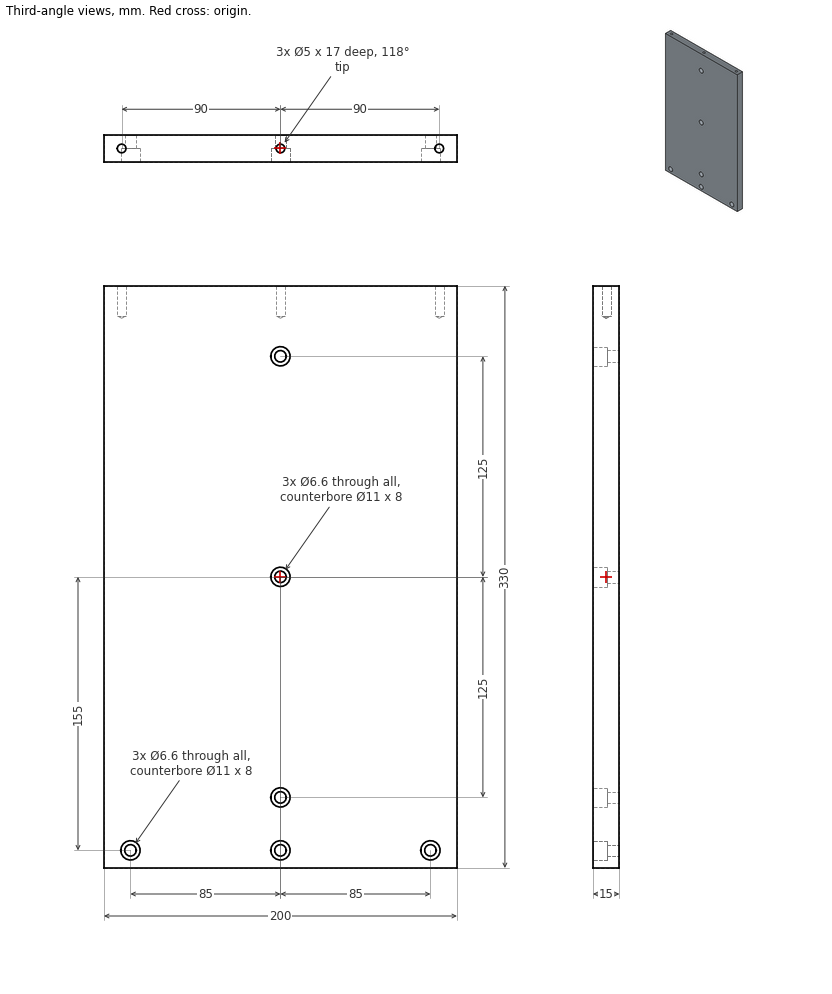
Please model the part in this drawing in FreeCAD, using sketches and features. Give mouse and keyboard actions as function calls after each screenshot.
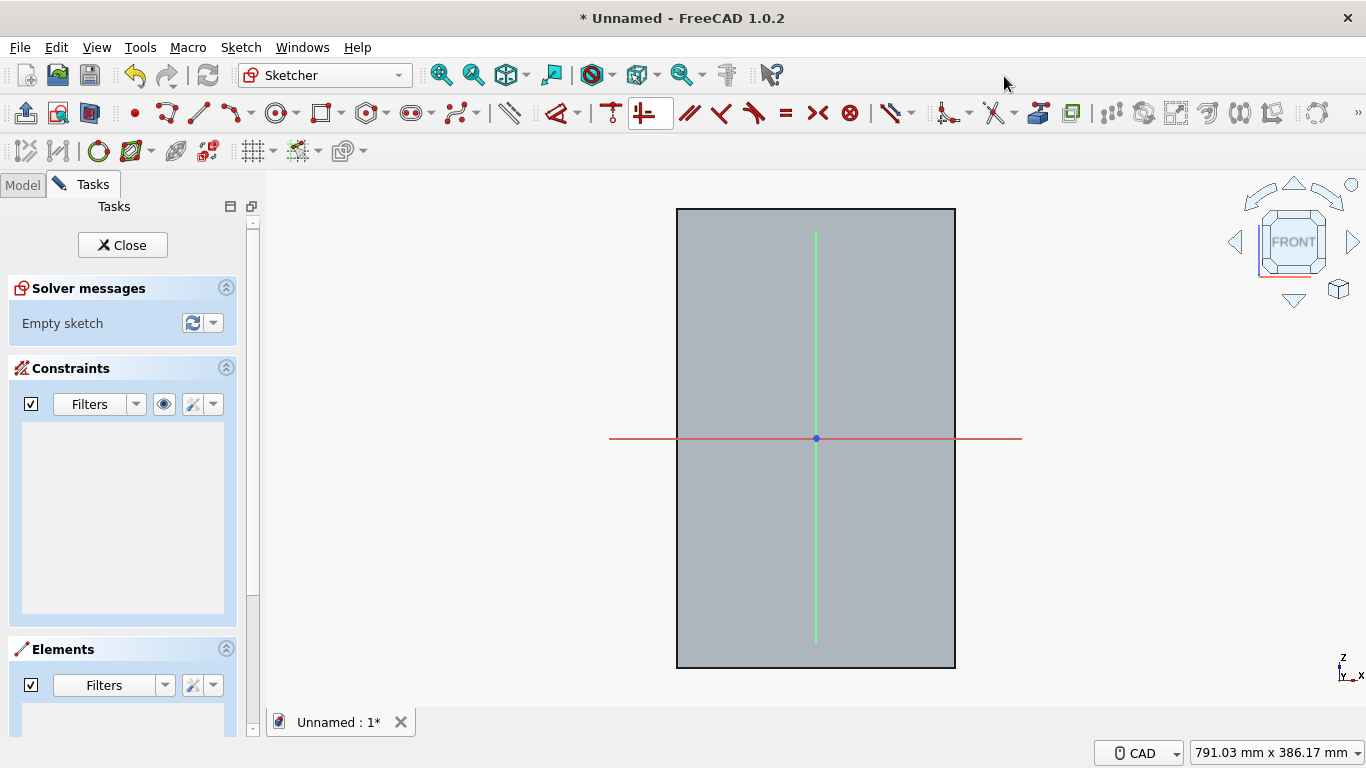
key(g)
key(c)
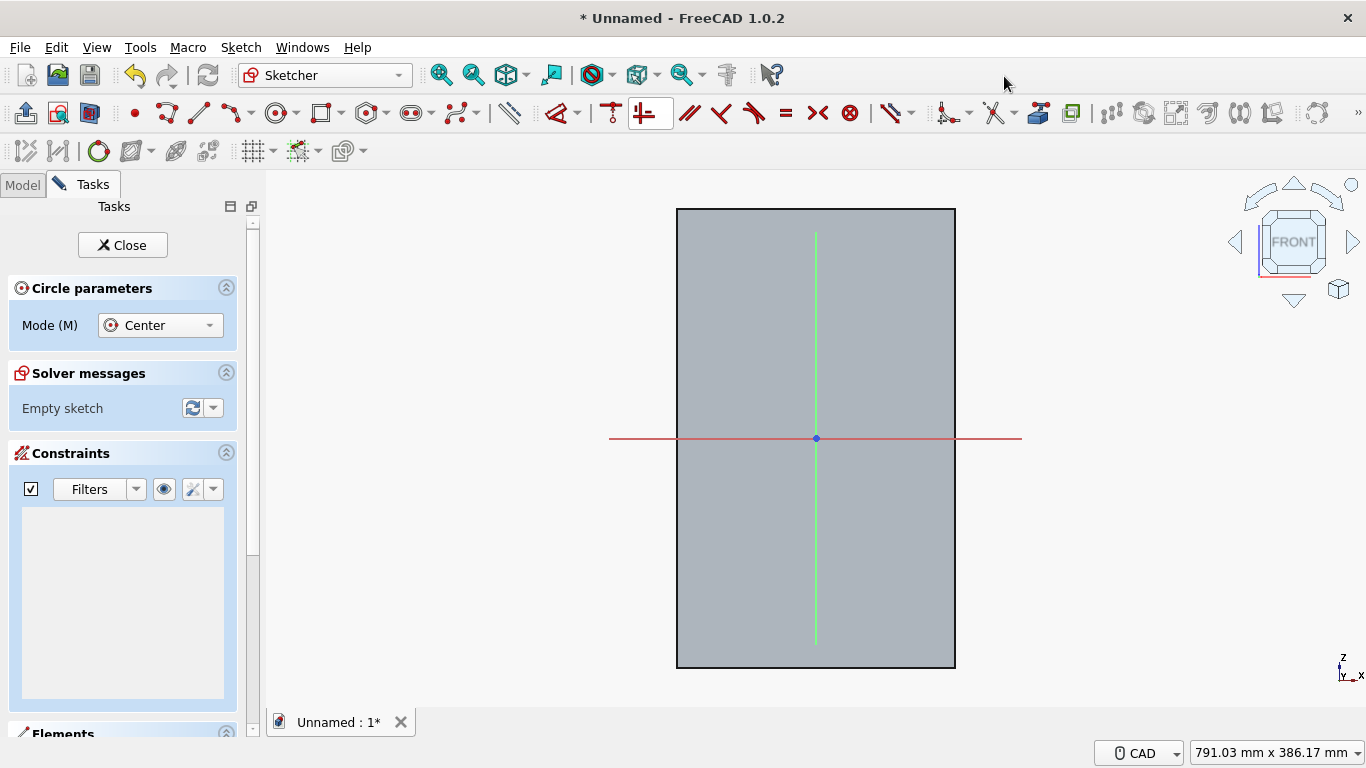
scroll(816, 439, up, 8)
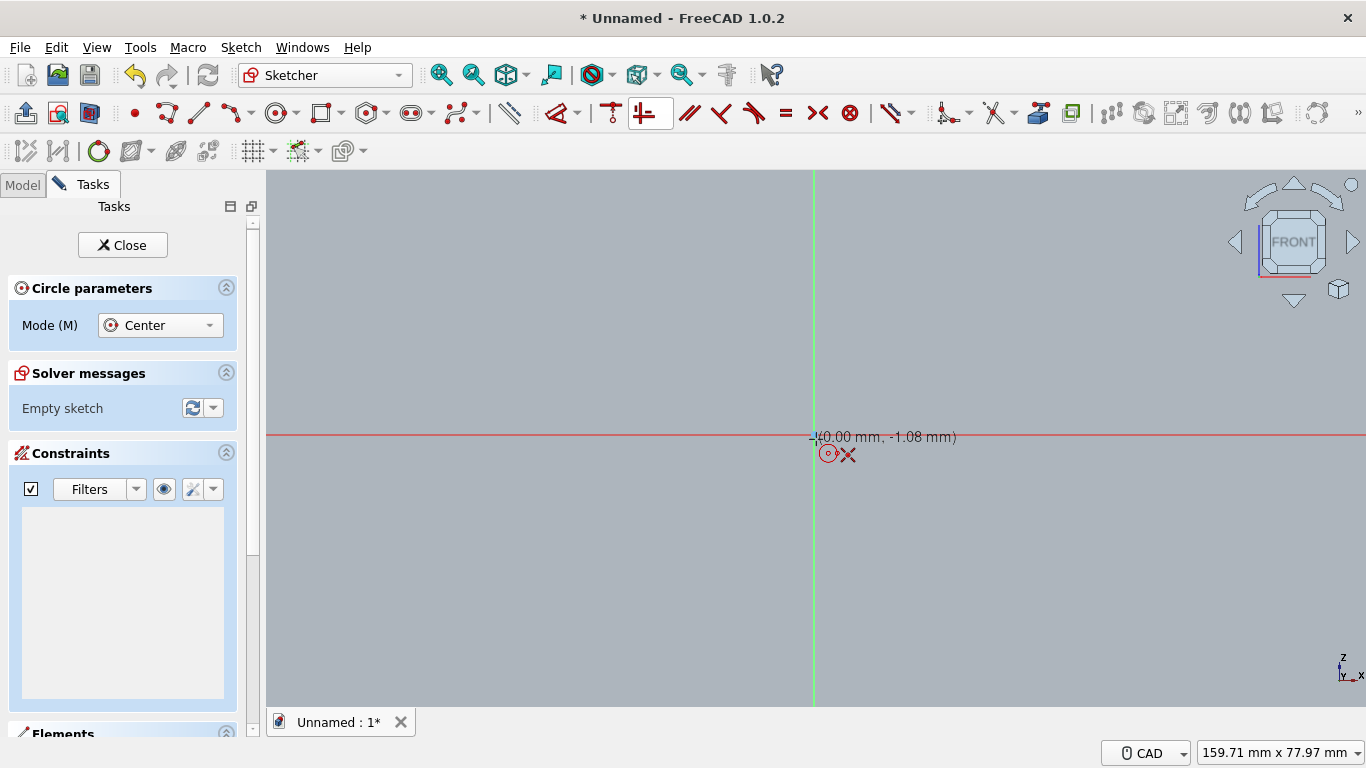
scroll(731, 440, down, 8)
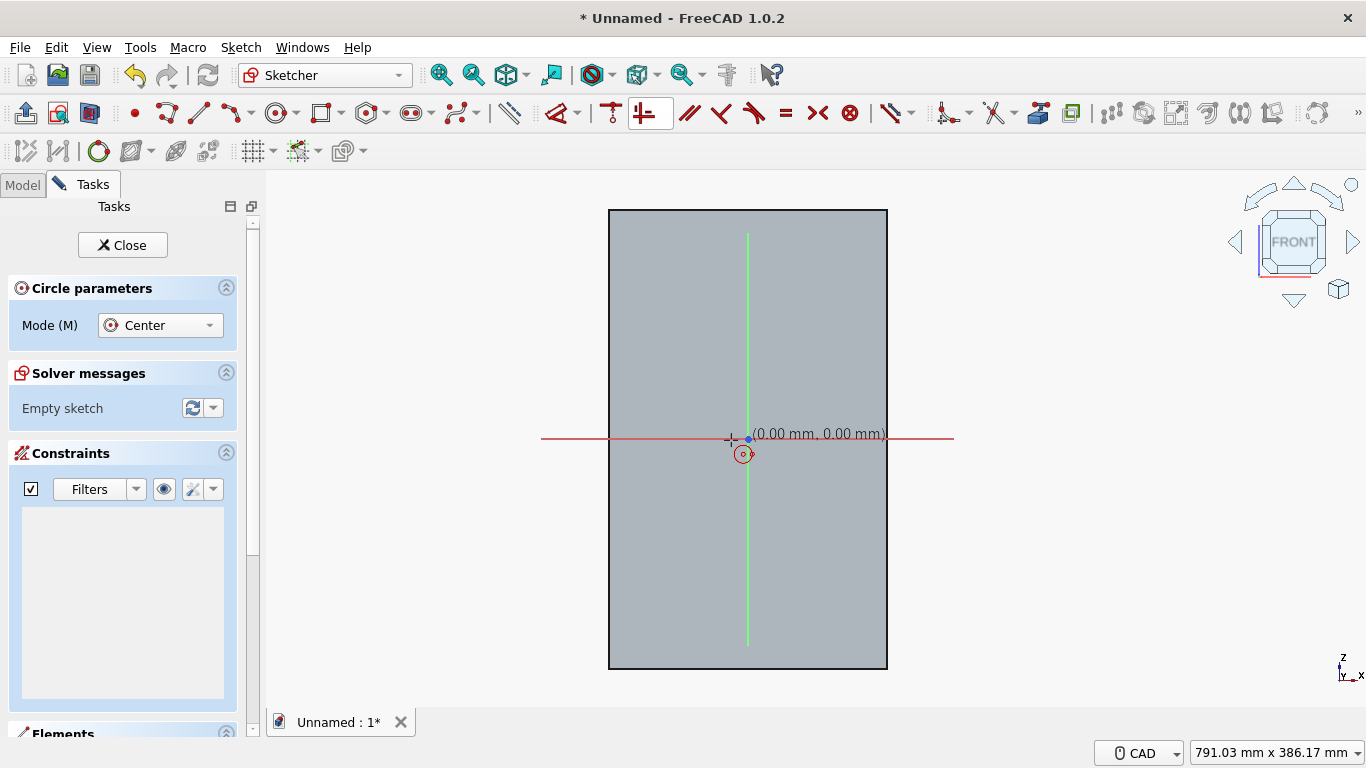
click(748, 439)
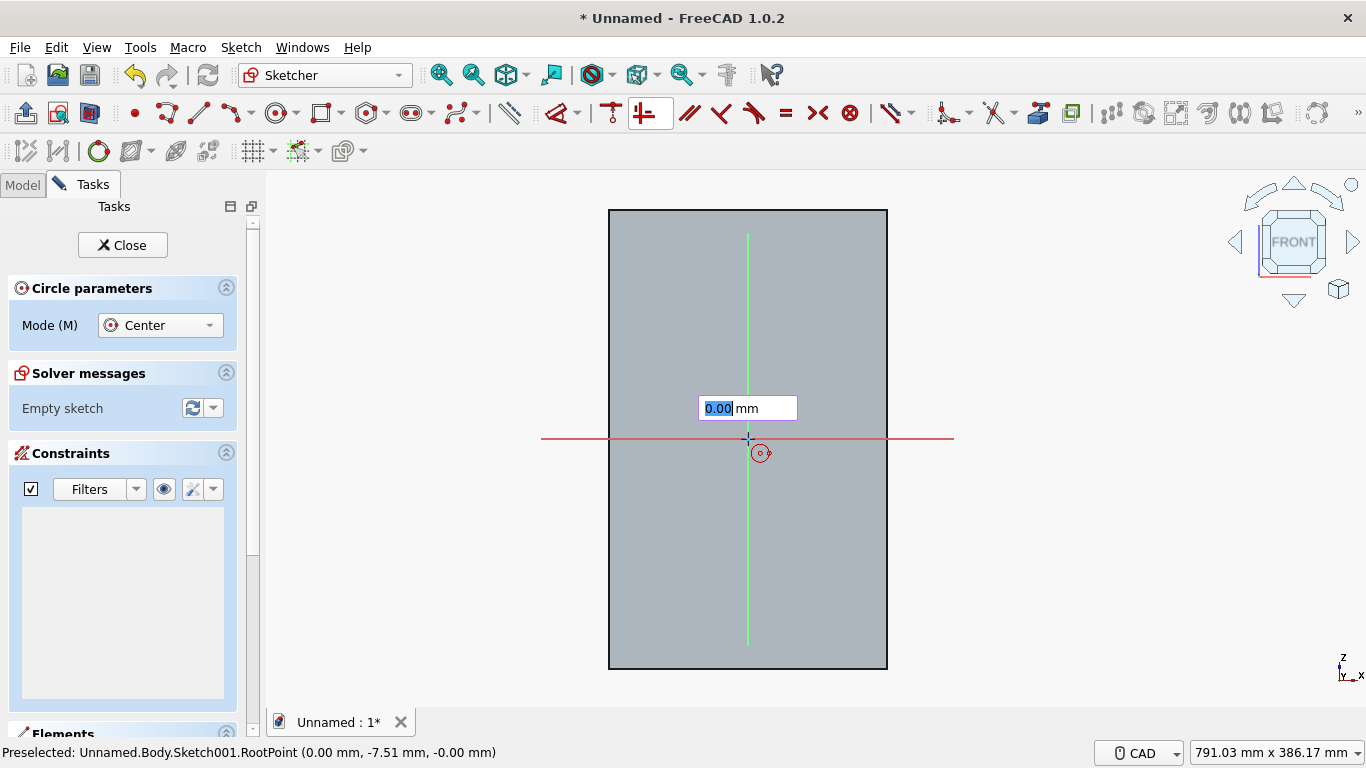
scroll(751, 436, up, 8)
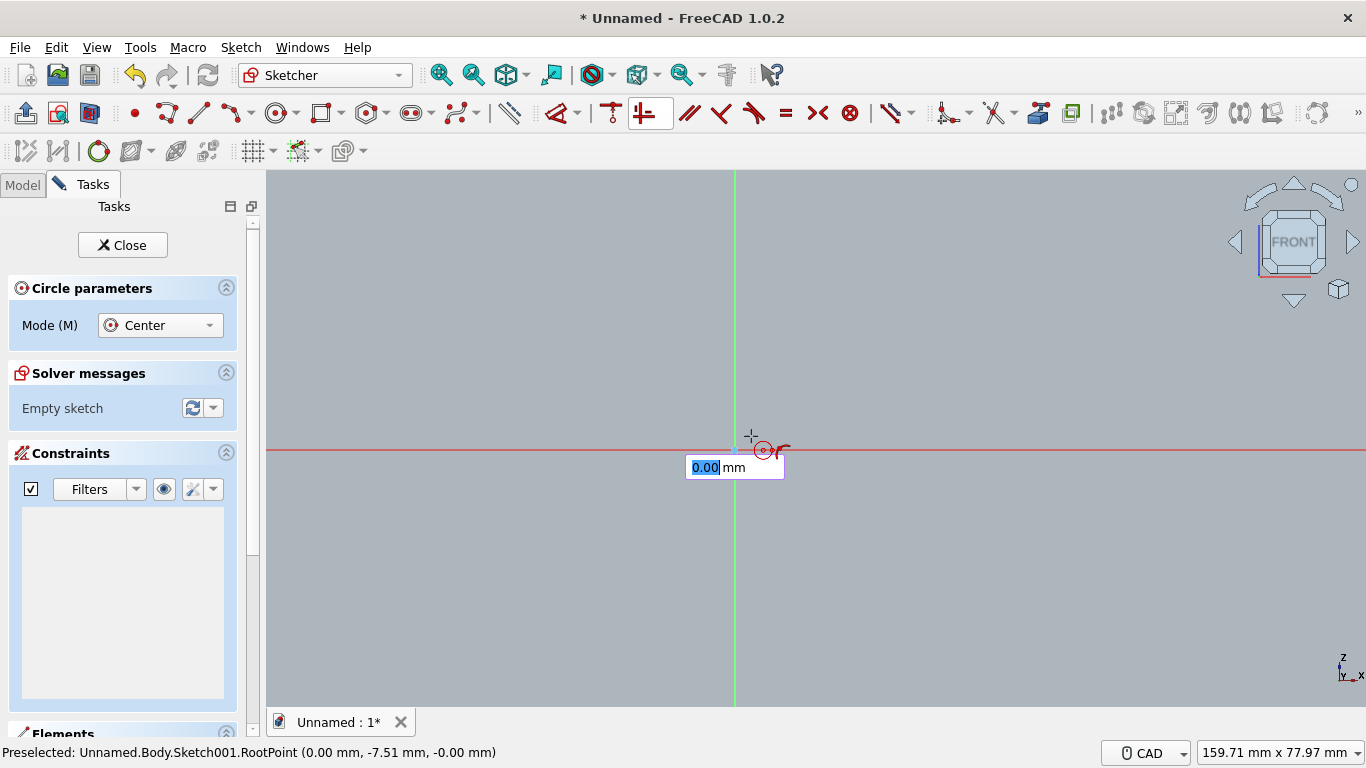
click(751, 434)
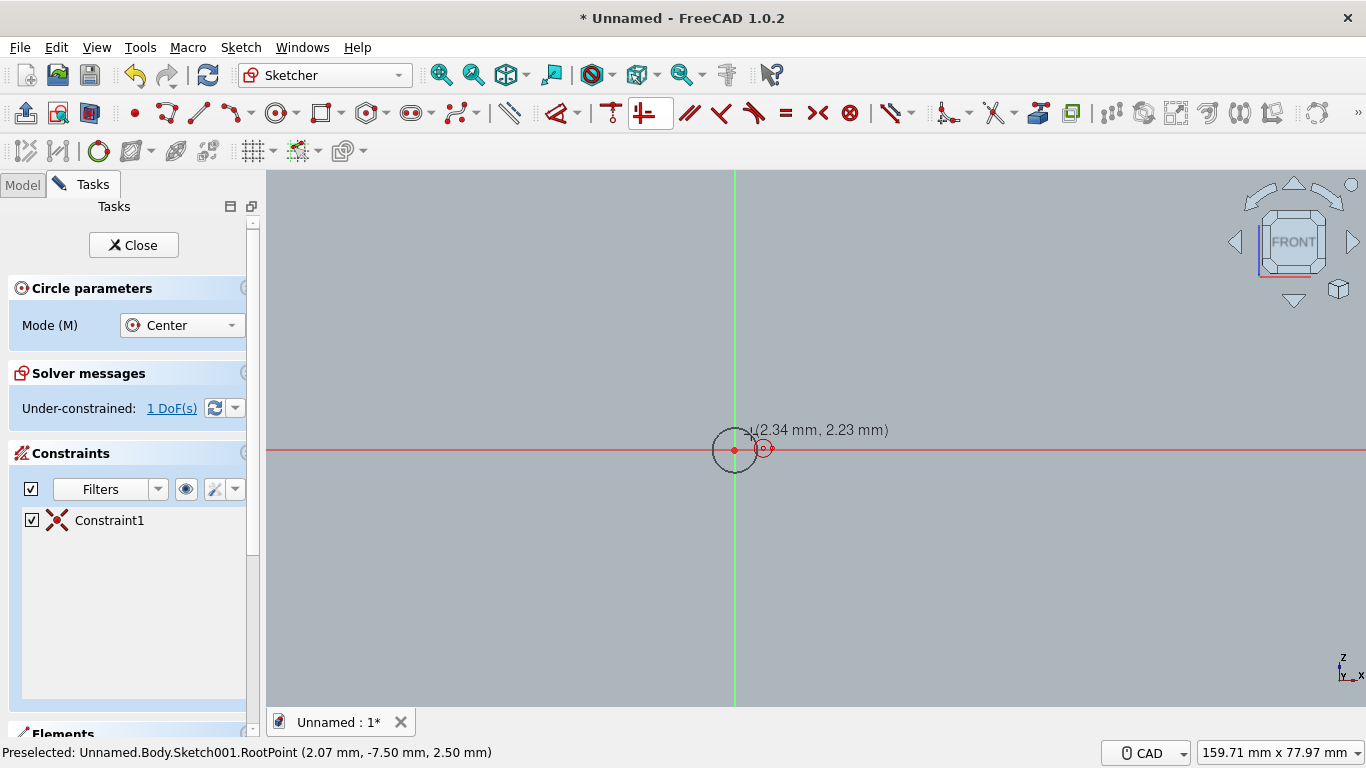
scroll(751, 435, down, 8)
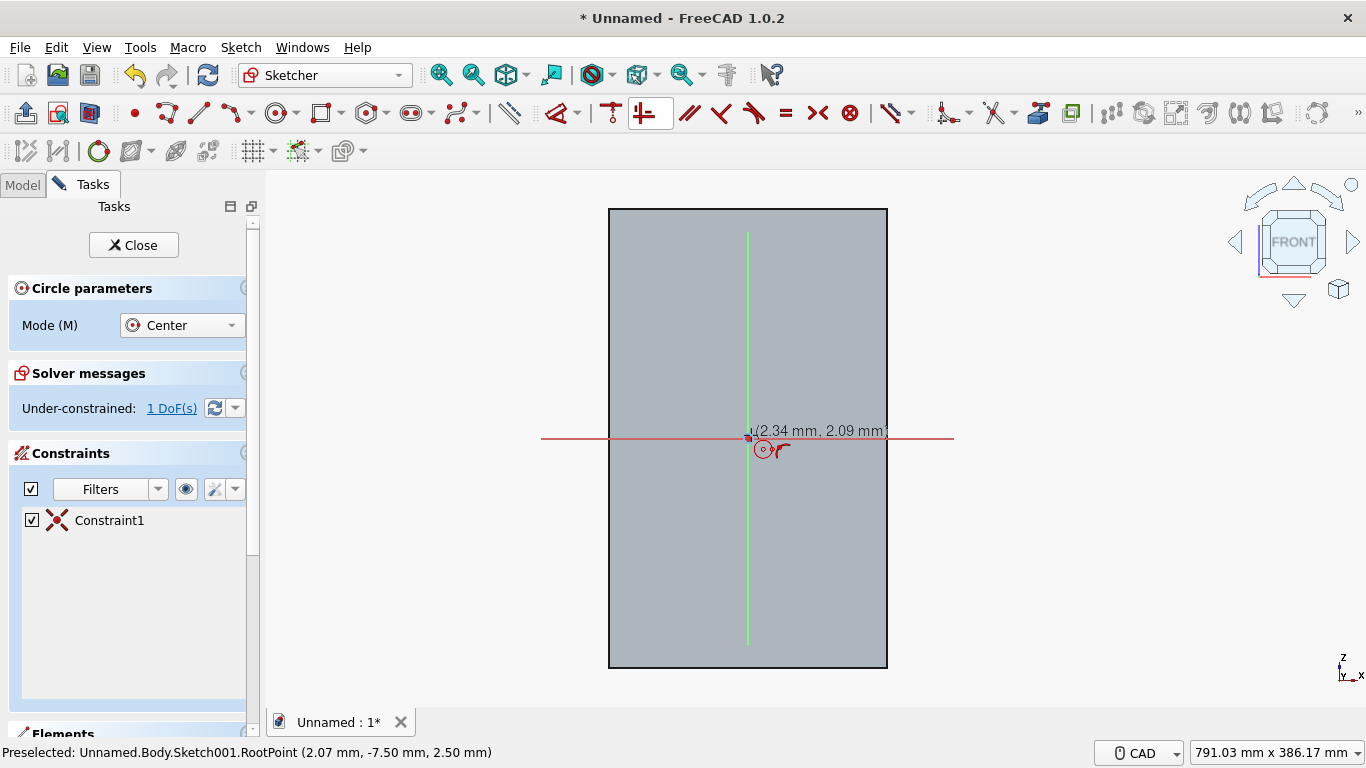
scroll(748, 265, up, 8)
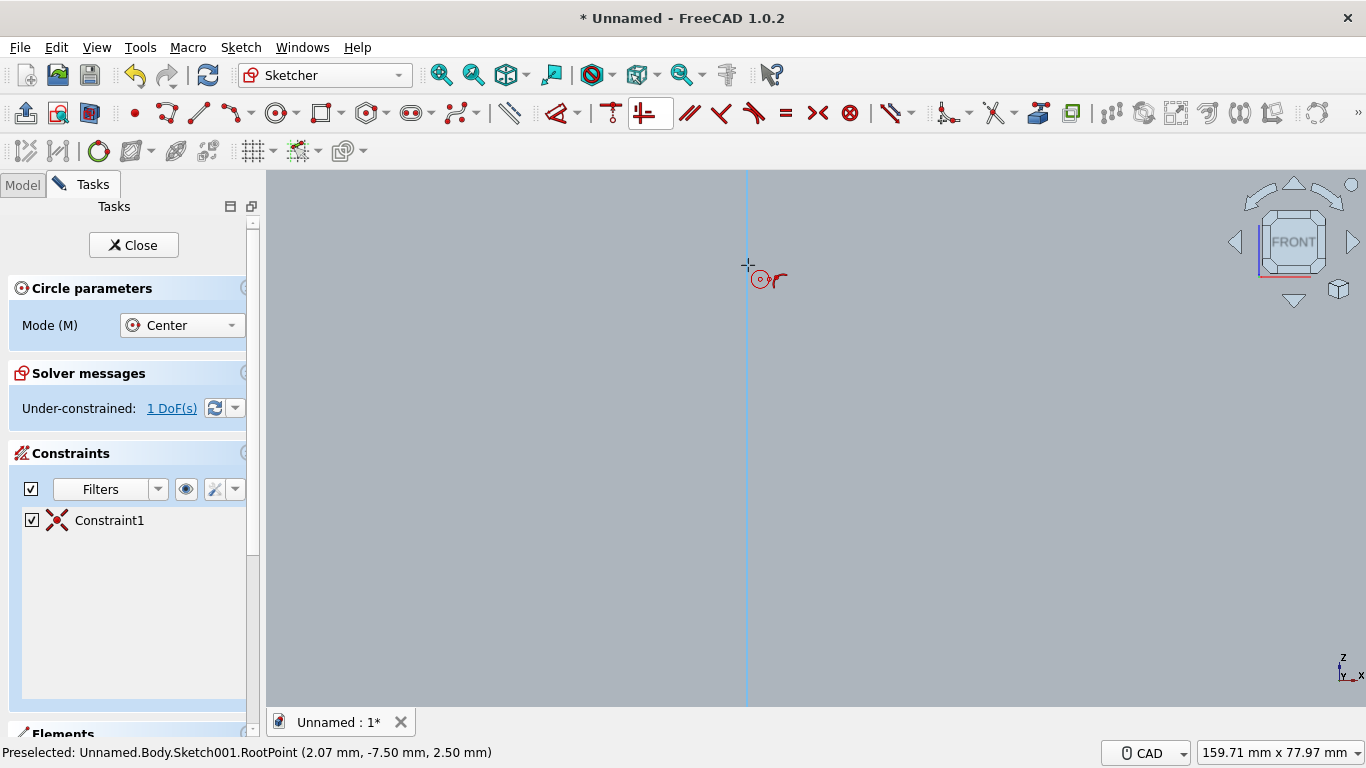
scroll(748, 265, down, 8)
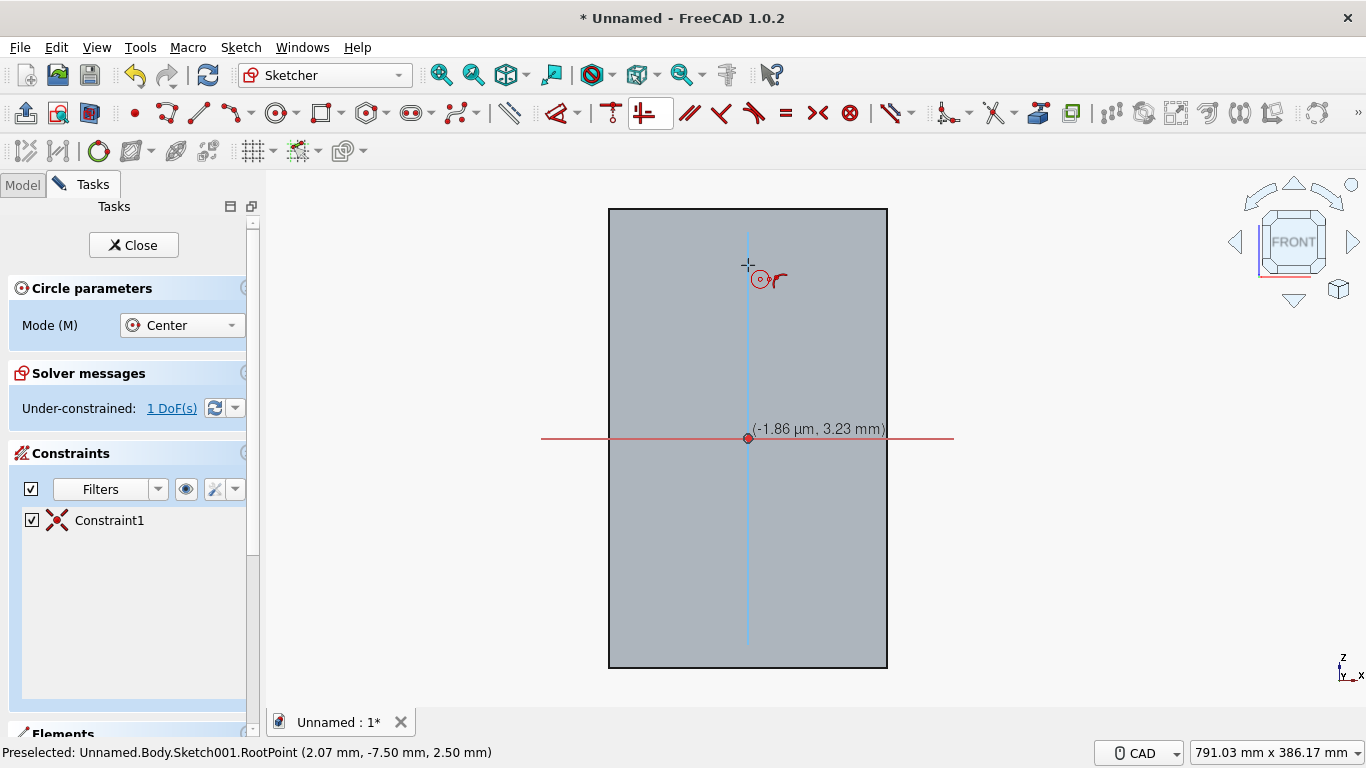
click(748, 265)